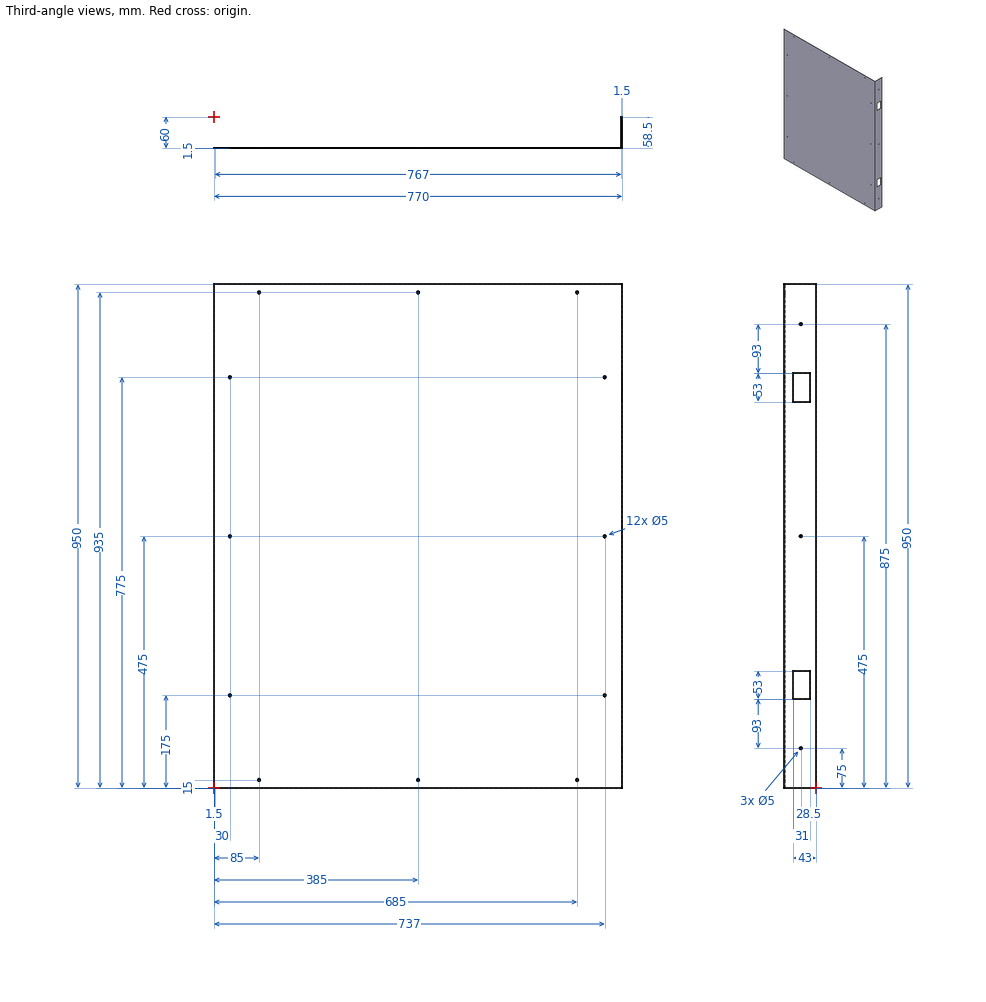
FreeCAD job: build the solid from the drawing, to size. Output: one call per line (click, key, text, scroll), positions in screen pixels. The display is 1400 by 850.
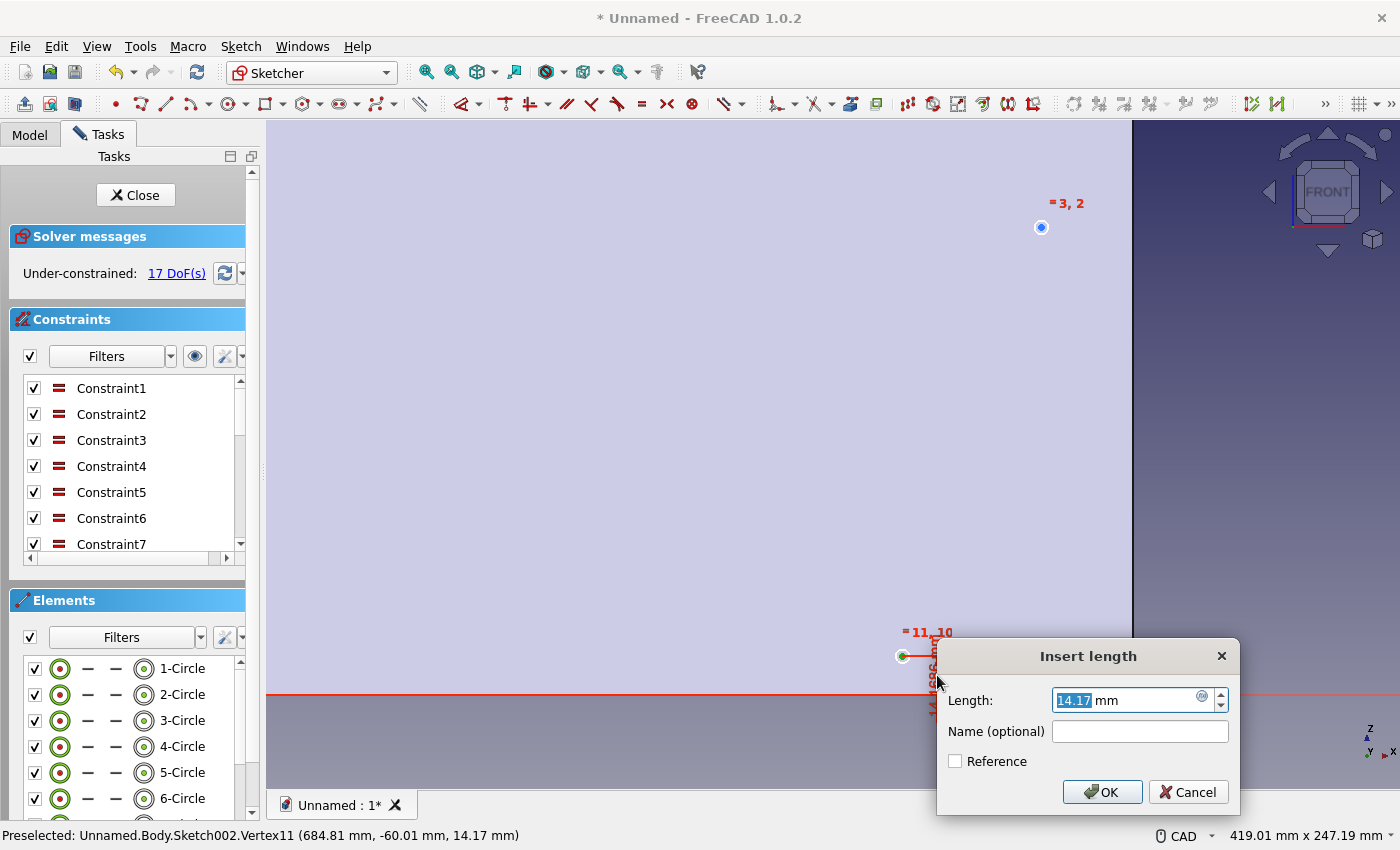
text(15)
key(Return)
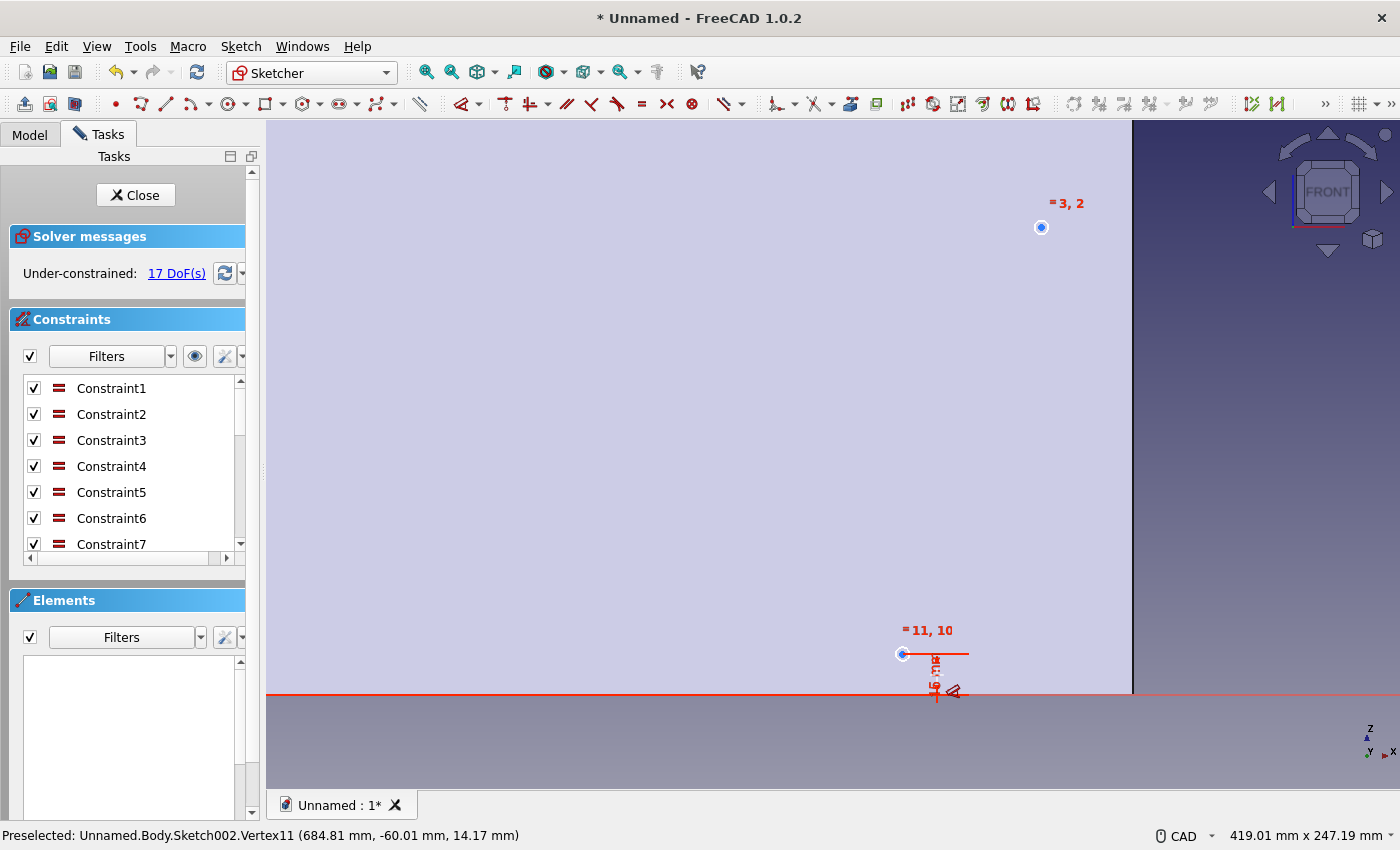
scroll(906, 658, down, 9)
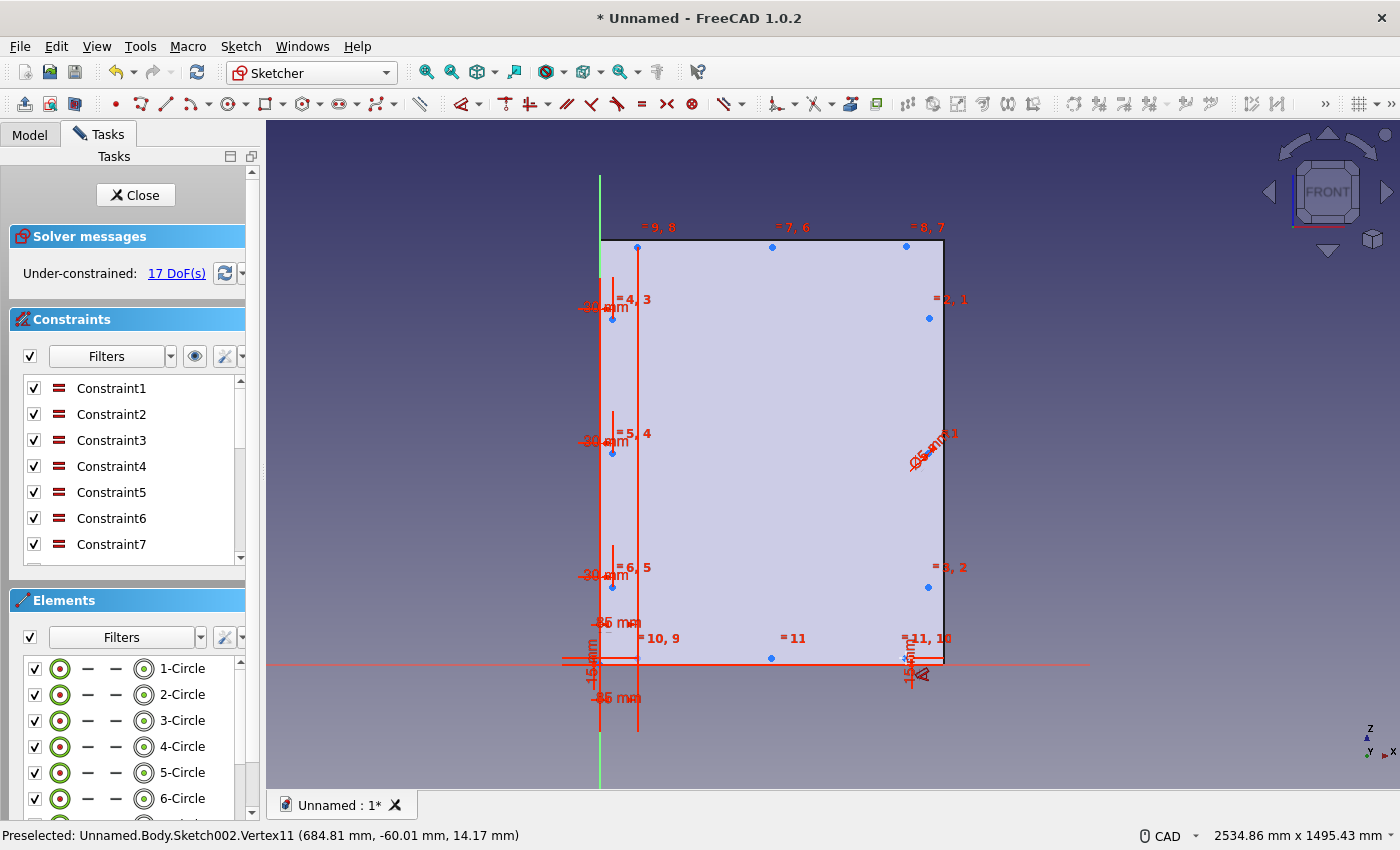
scroll(772, 658, up, 9)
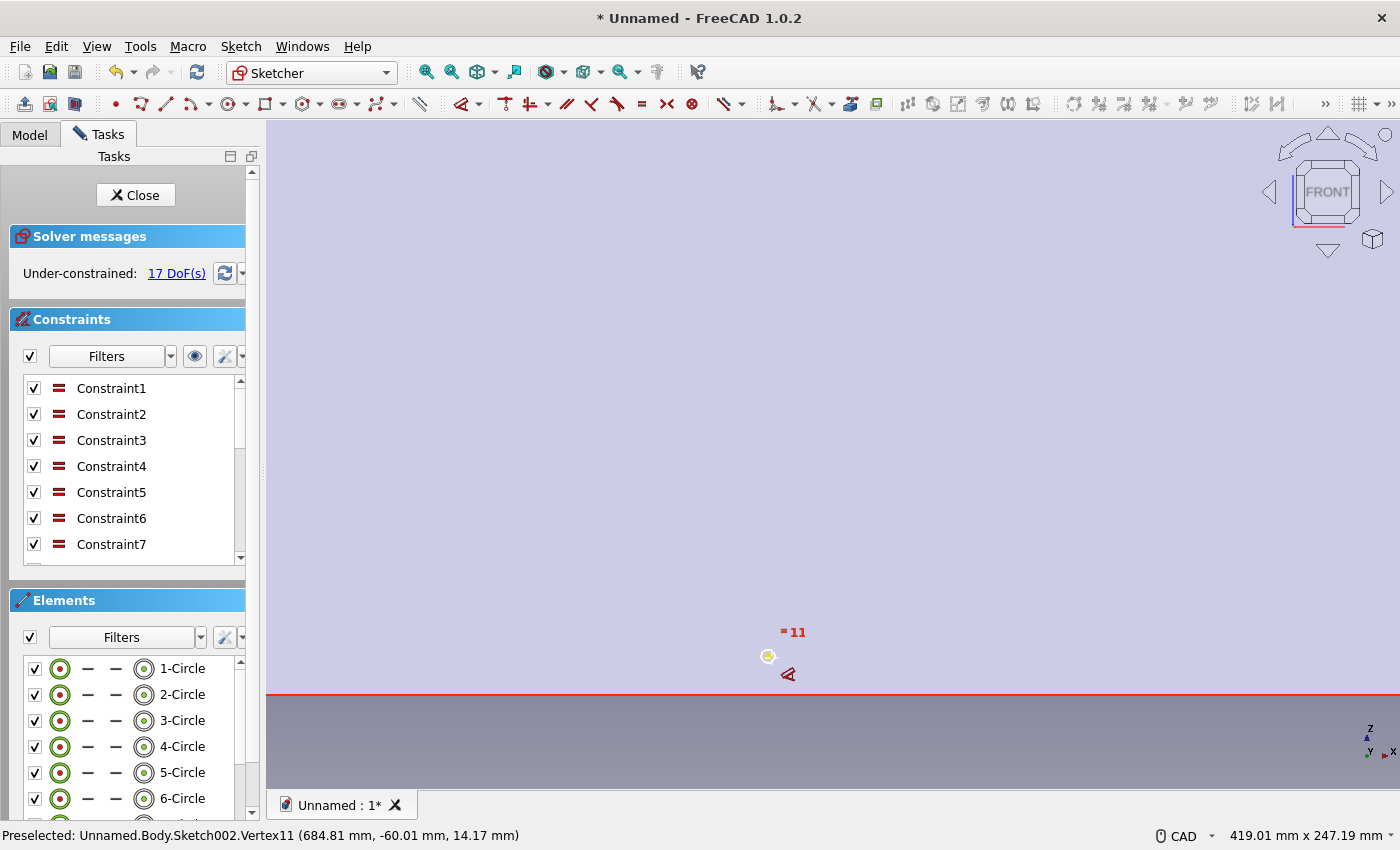
click(768, 656)
click(802, 675)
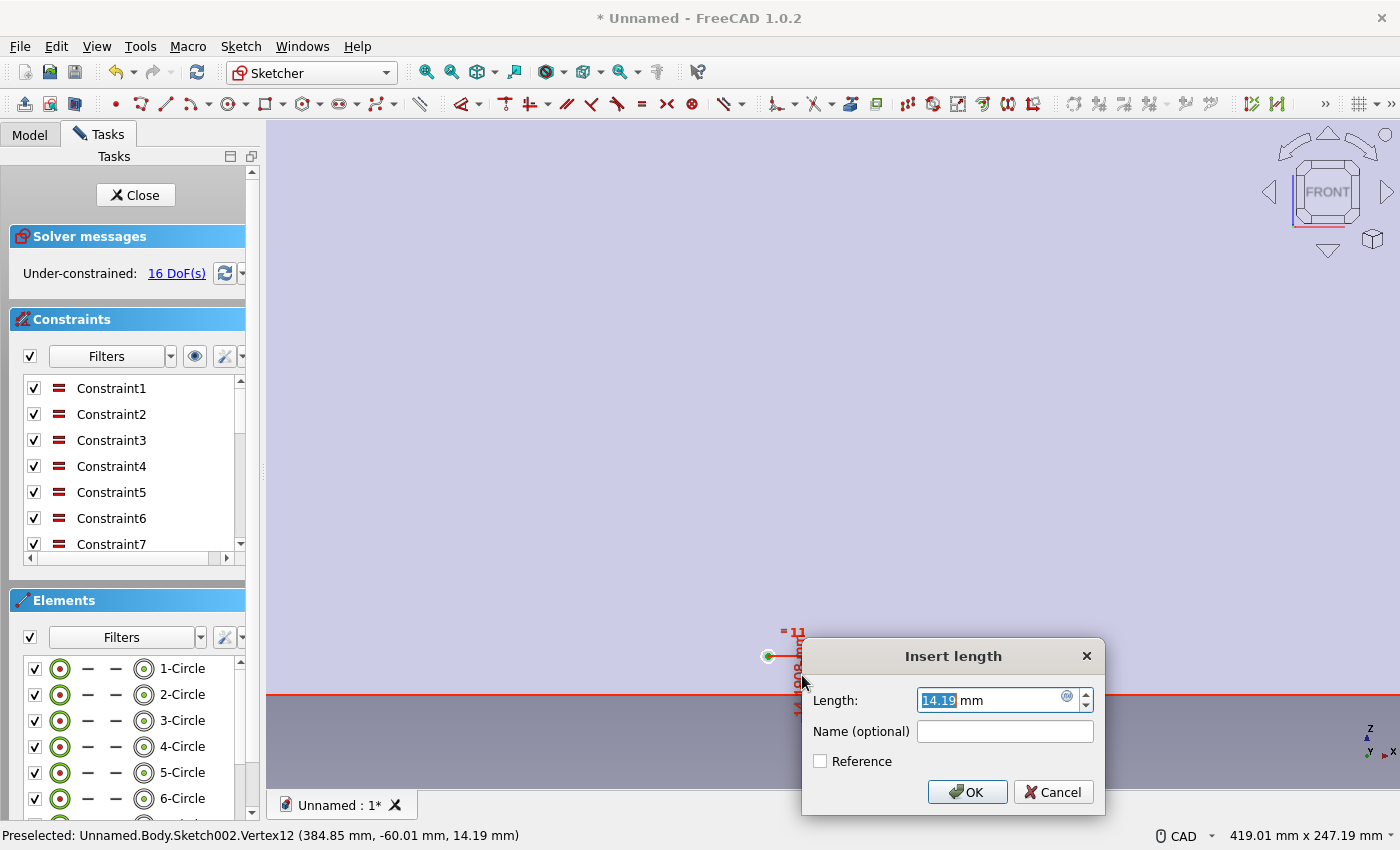
text(15)
key(Return)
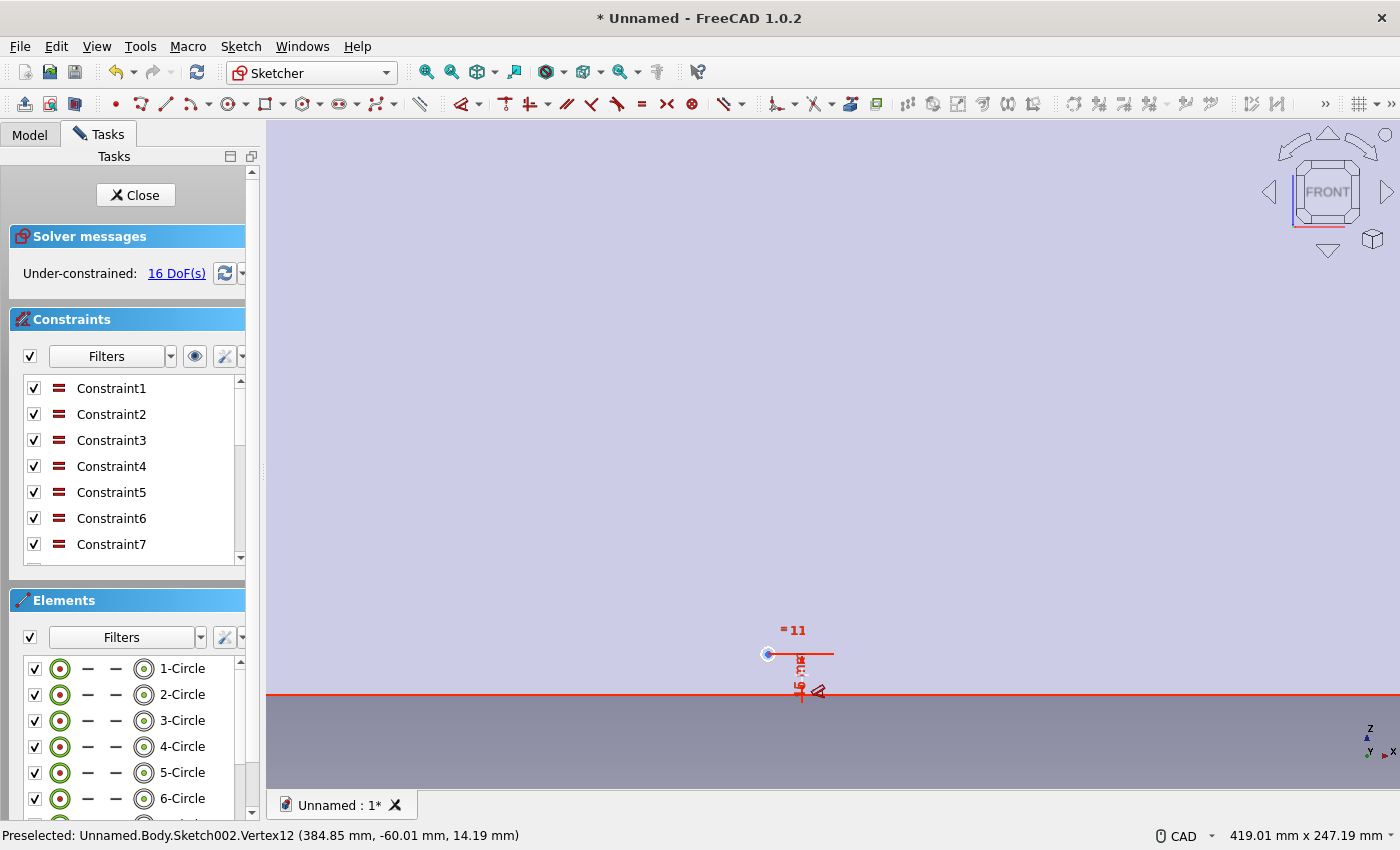
scroll(772, 658, down, 9)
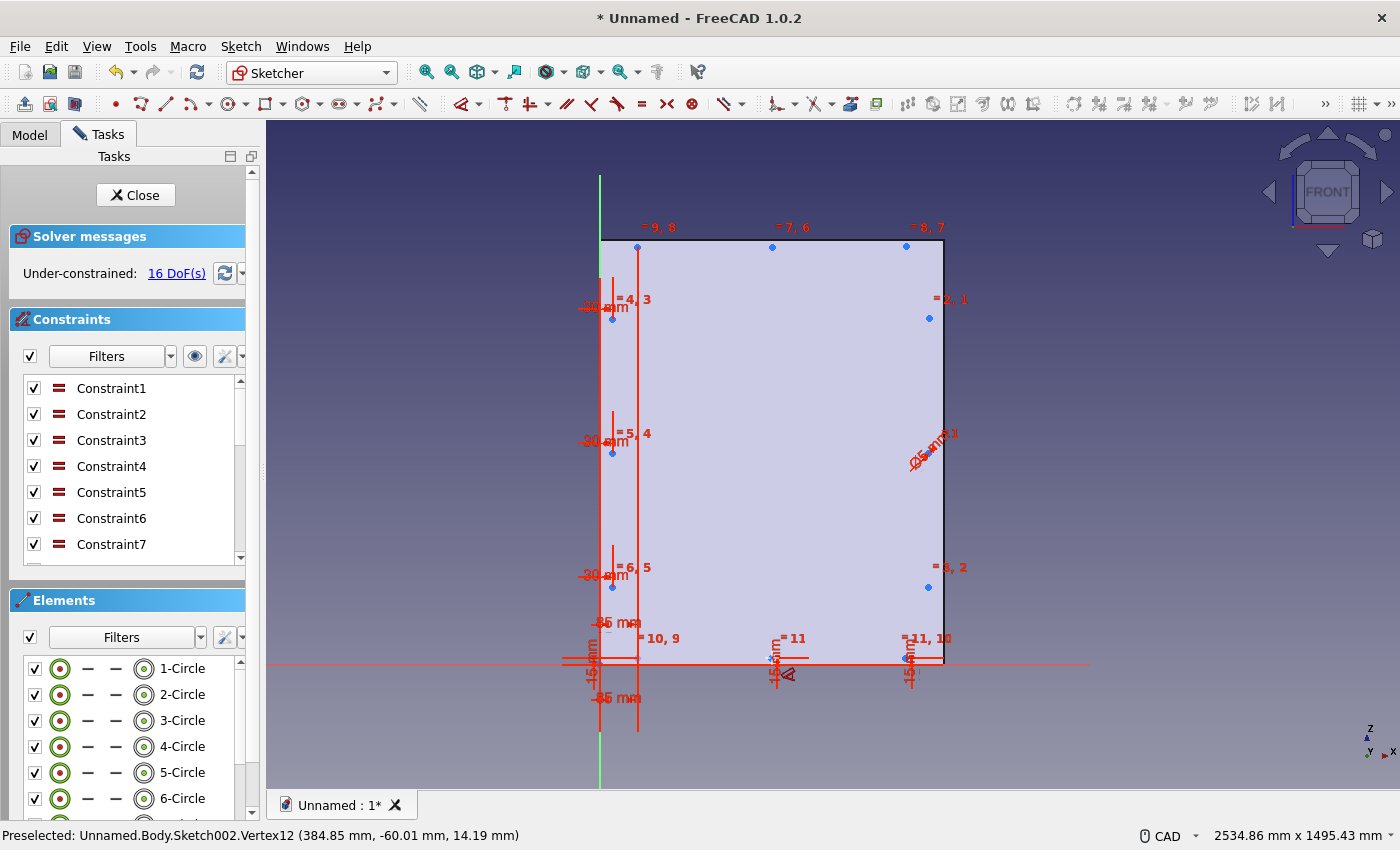
click(929, 453)
click(764, 699)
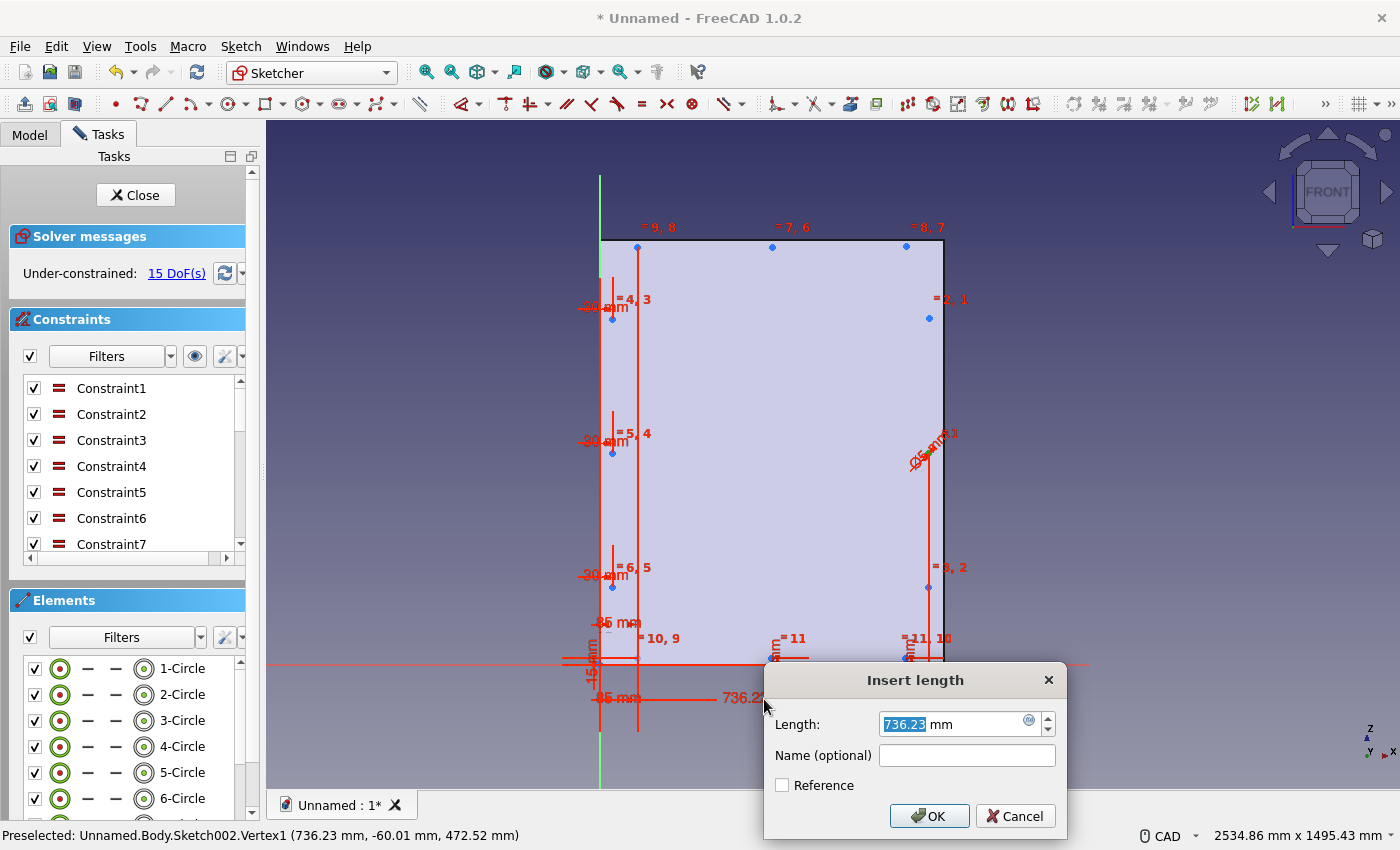
text(737)
key(Return)